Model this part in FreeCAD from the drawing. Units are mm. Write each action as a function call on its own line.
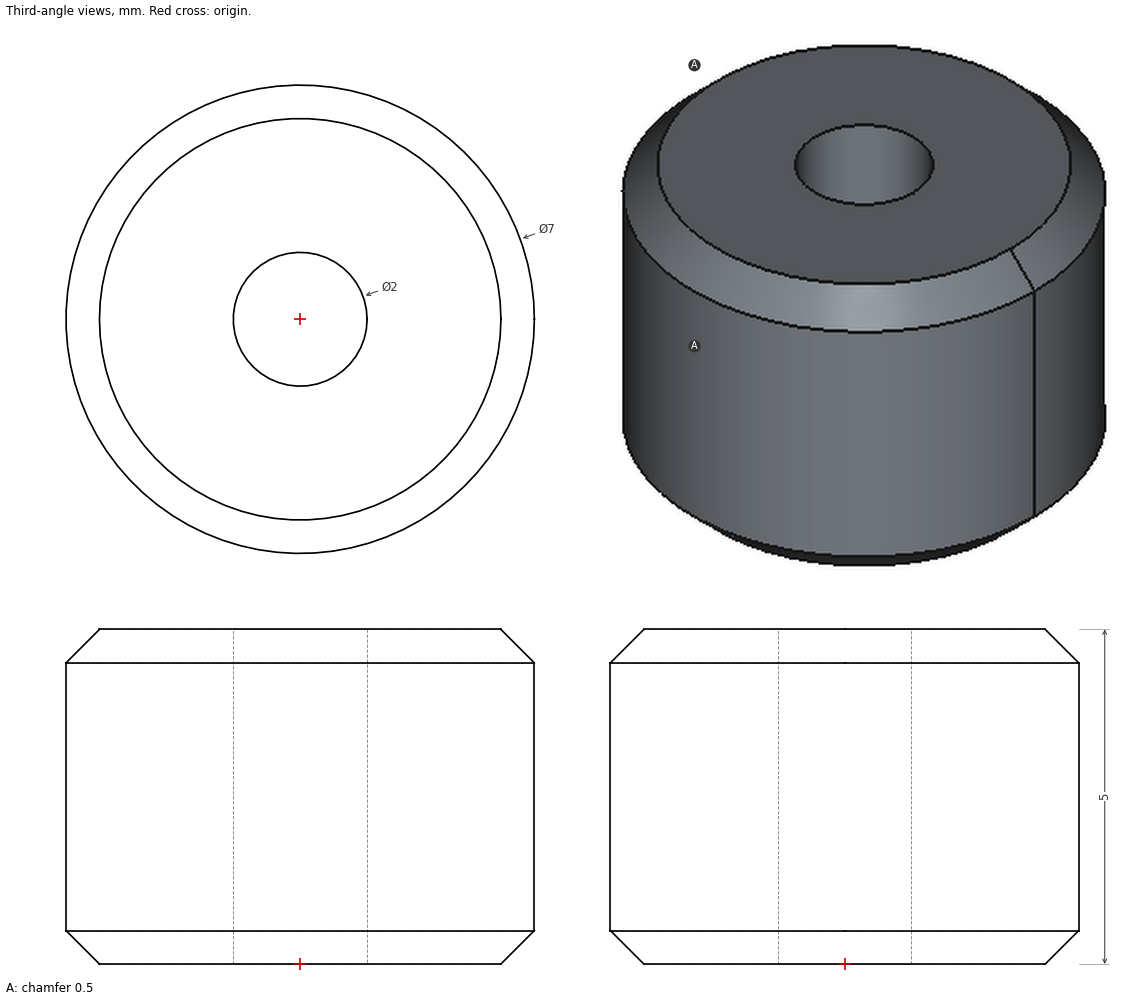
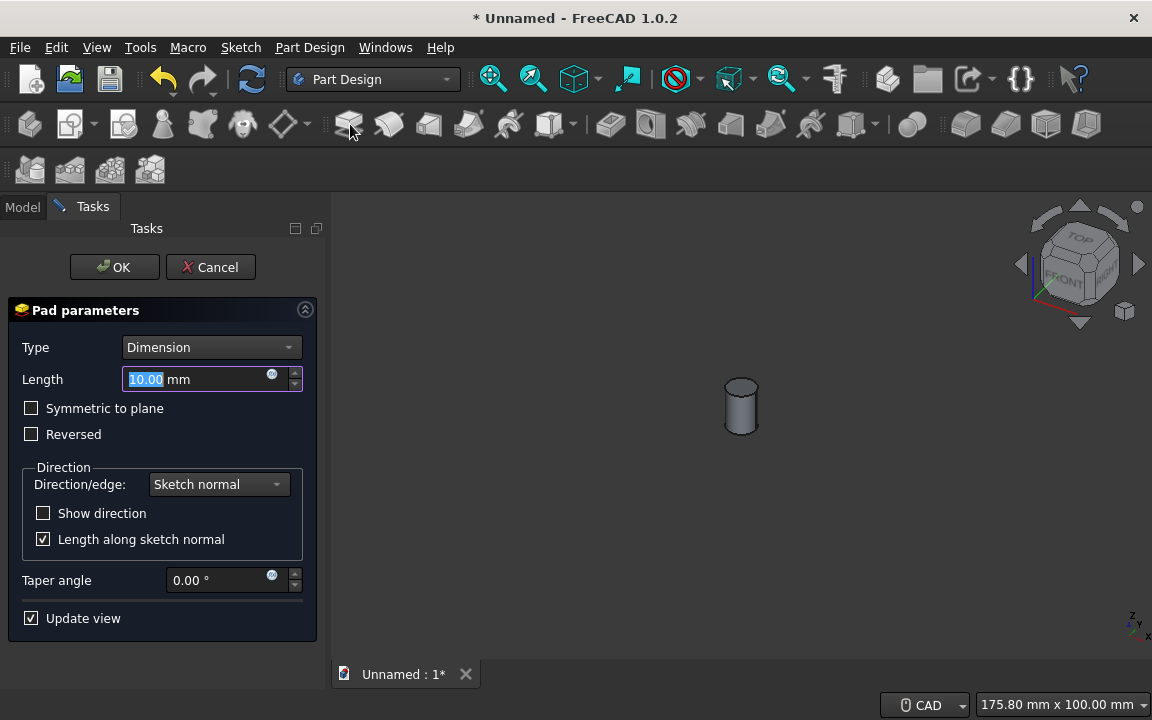
text(5)
key(Tab)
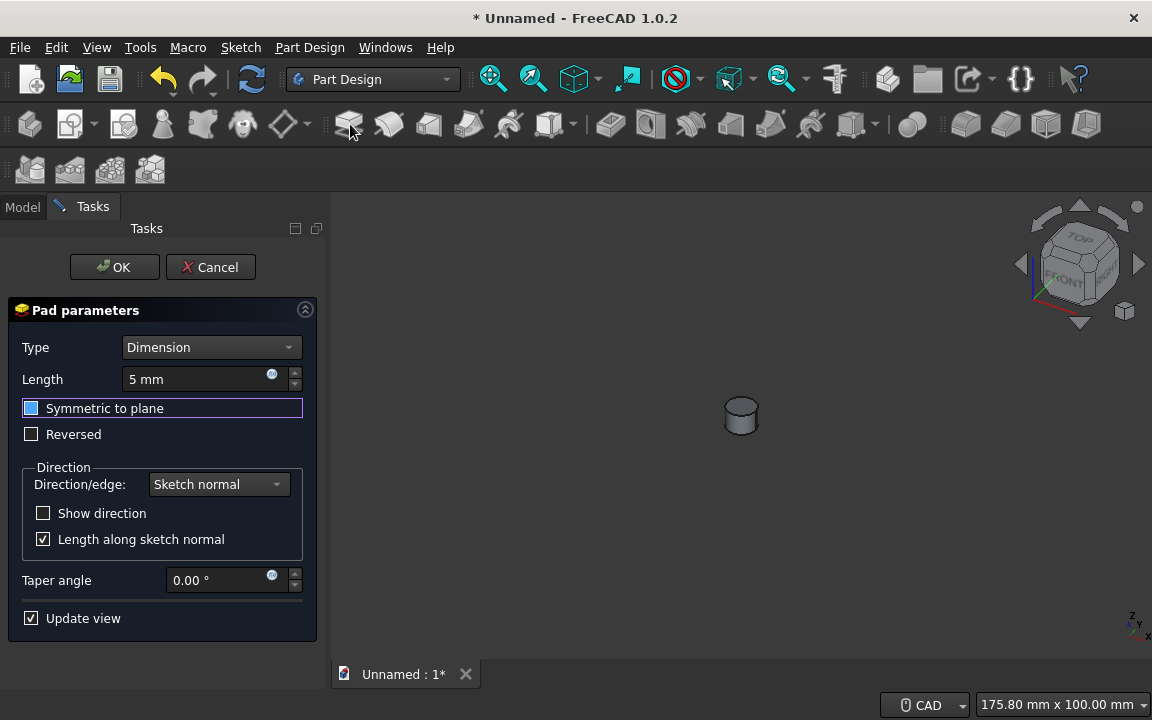
click(115, 267)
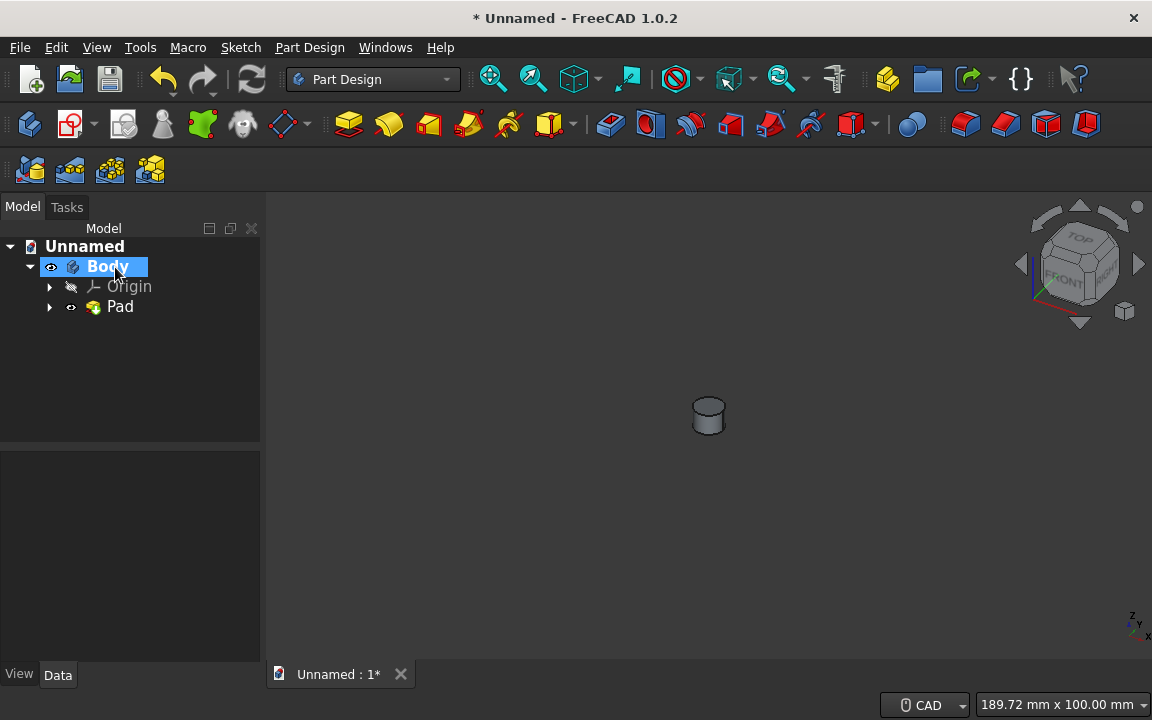
click(494, 80)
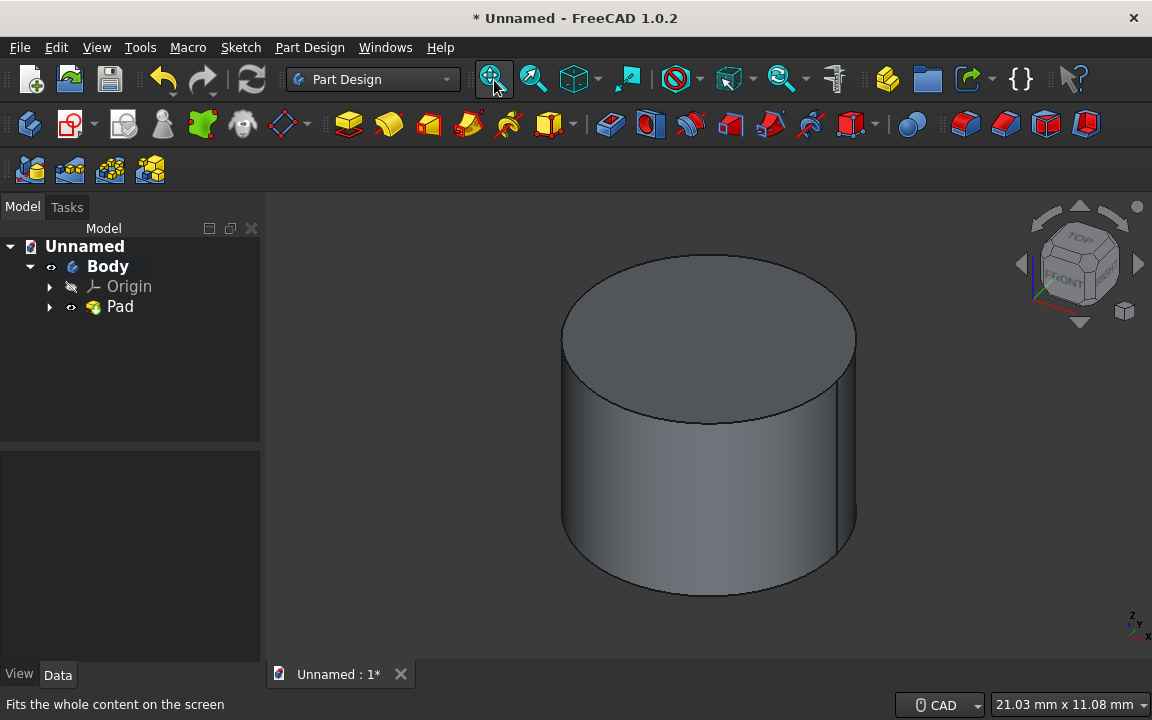
click(709, 338)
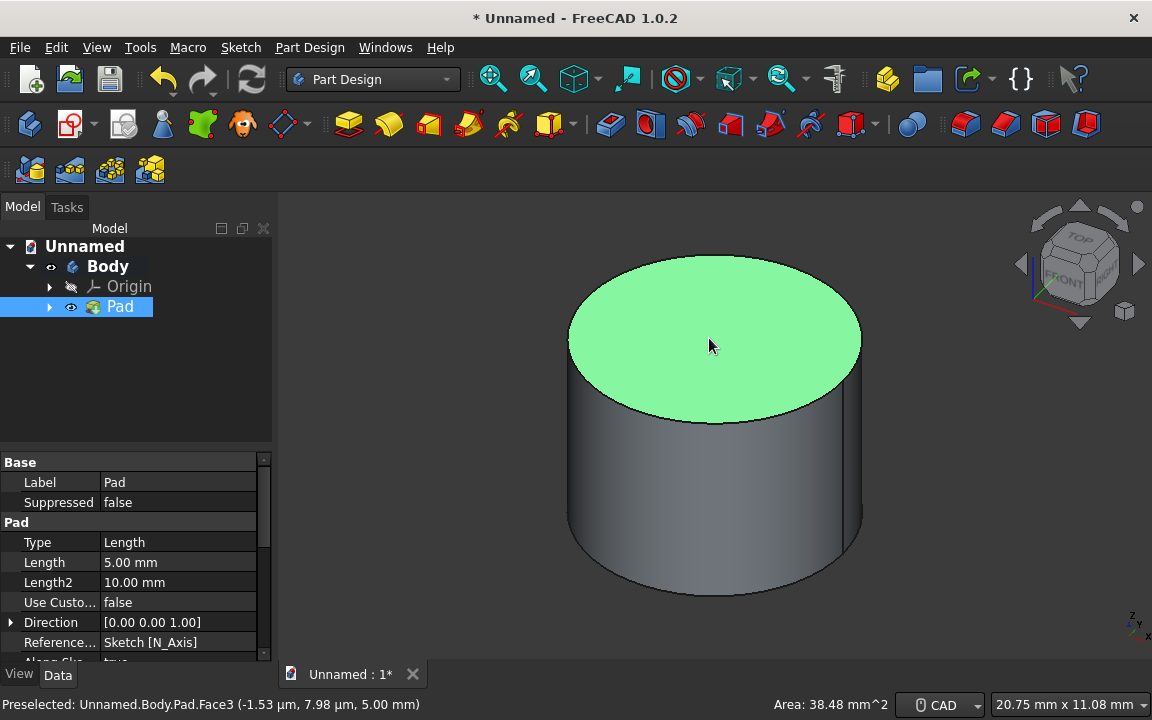
click(70, 124)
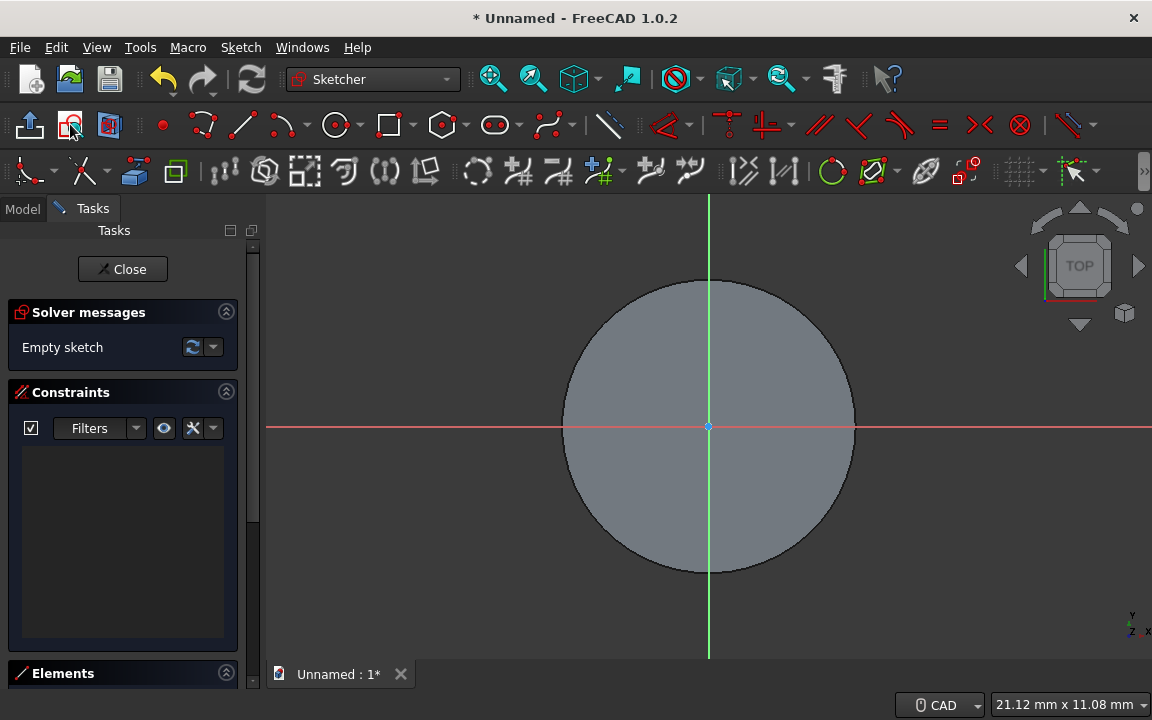
scroll(738, 427, up, 6)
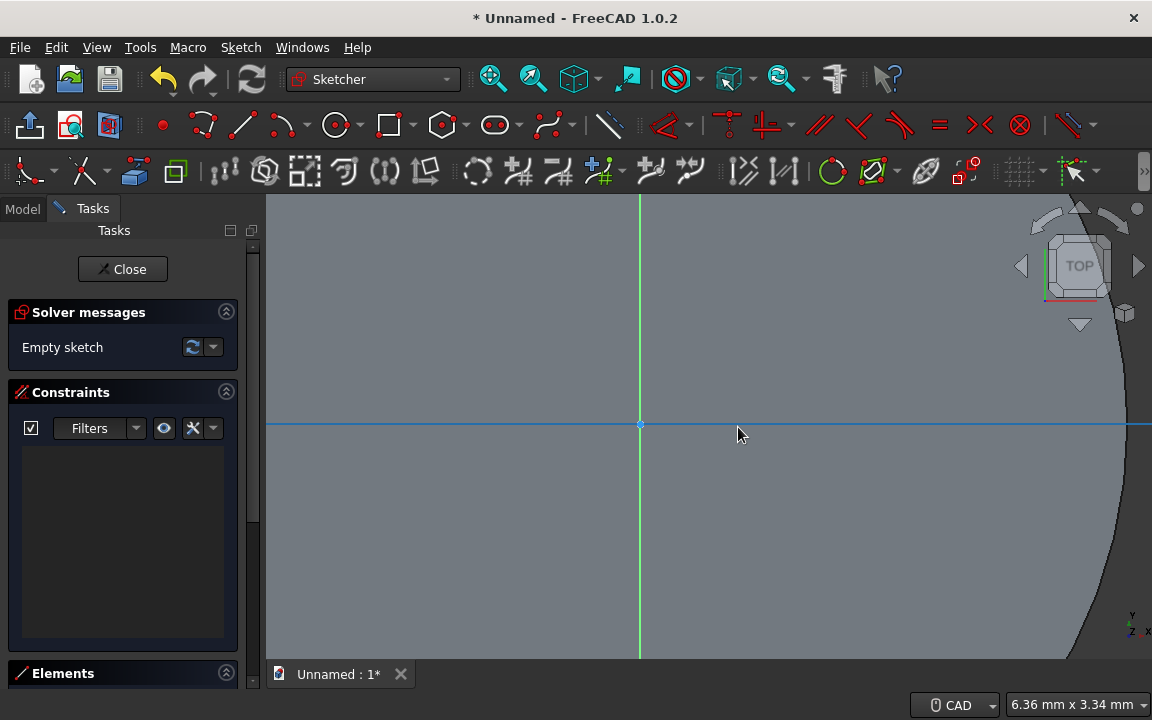
click(336, 126)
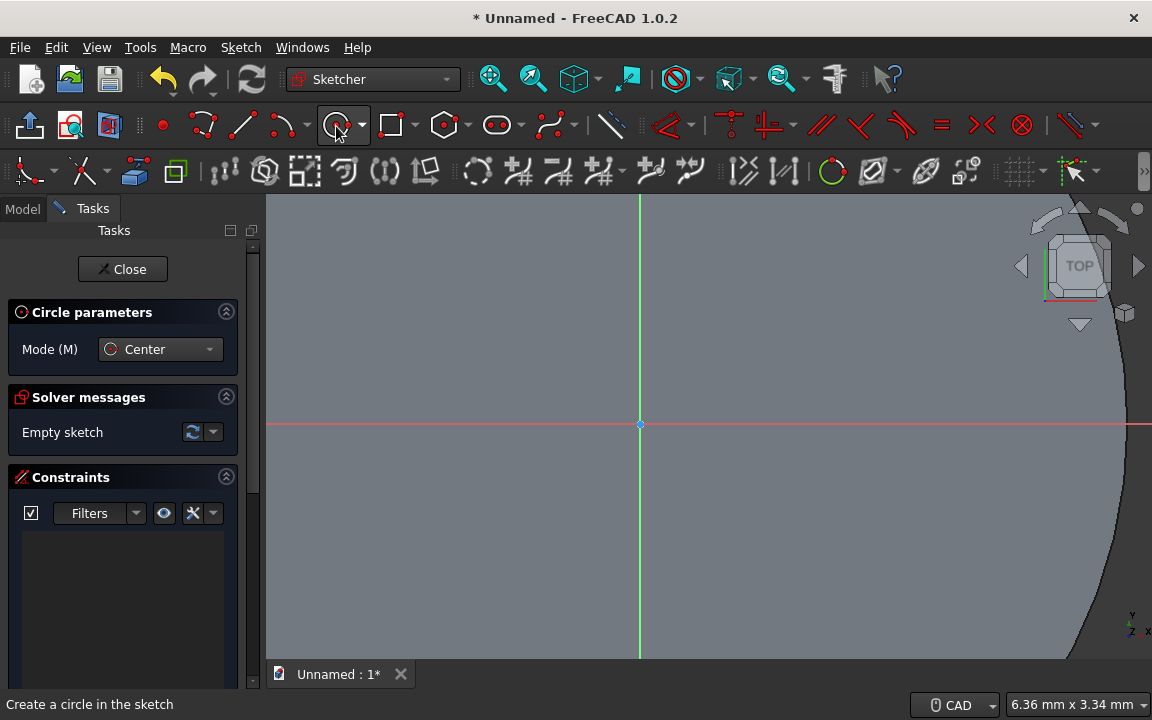
click(640, 424)
click(739, 326)
key(Escape)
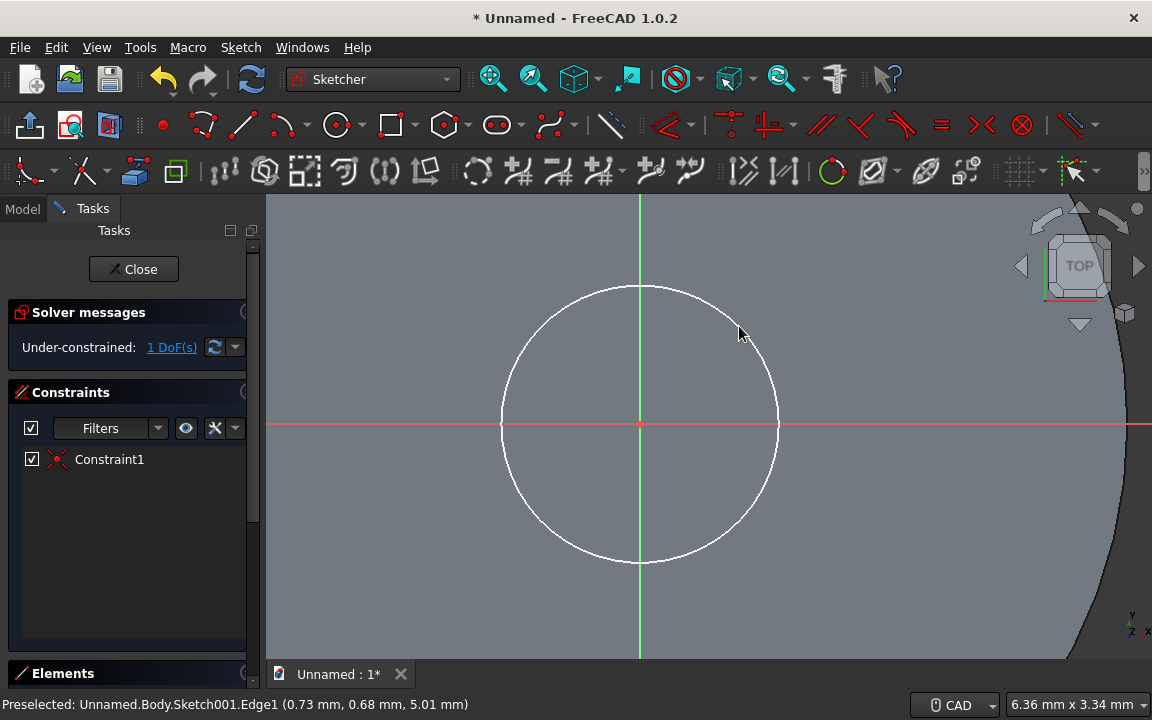
click(666, 126)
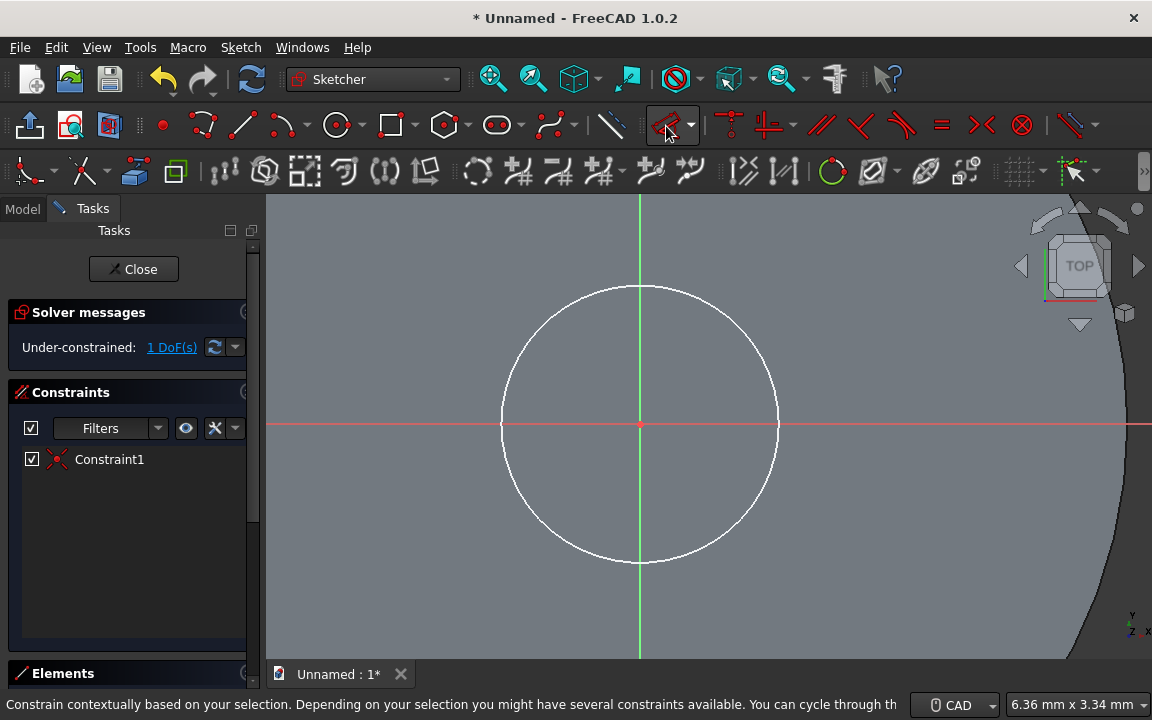
click(738, 326)
click(761, 303)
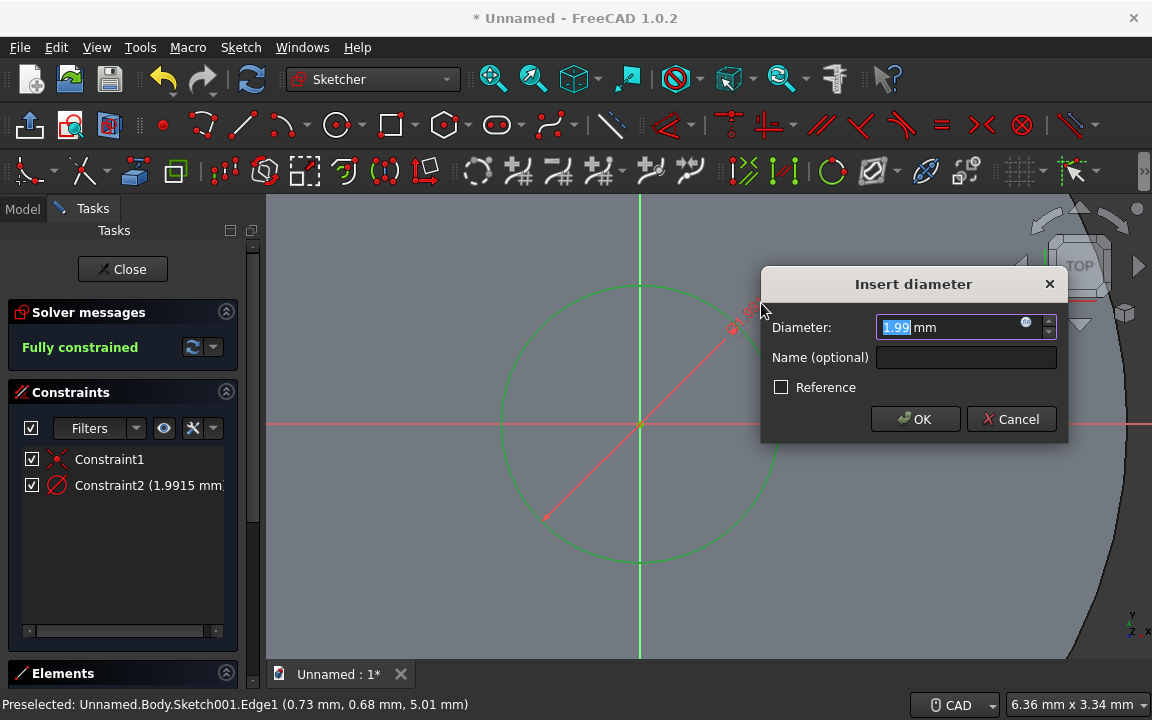
text(2)
key(Return)
key(Escape)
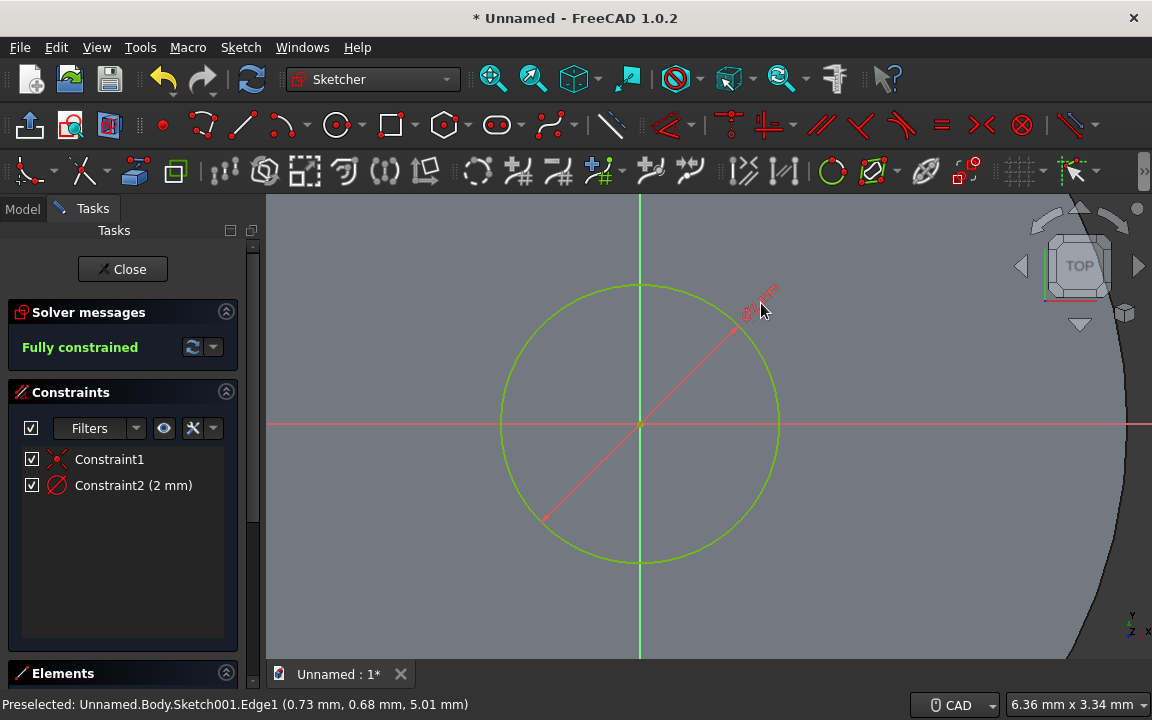
click(123, 269)